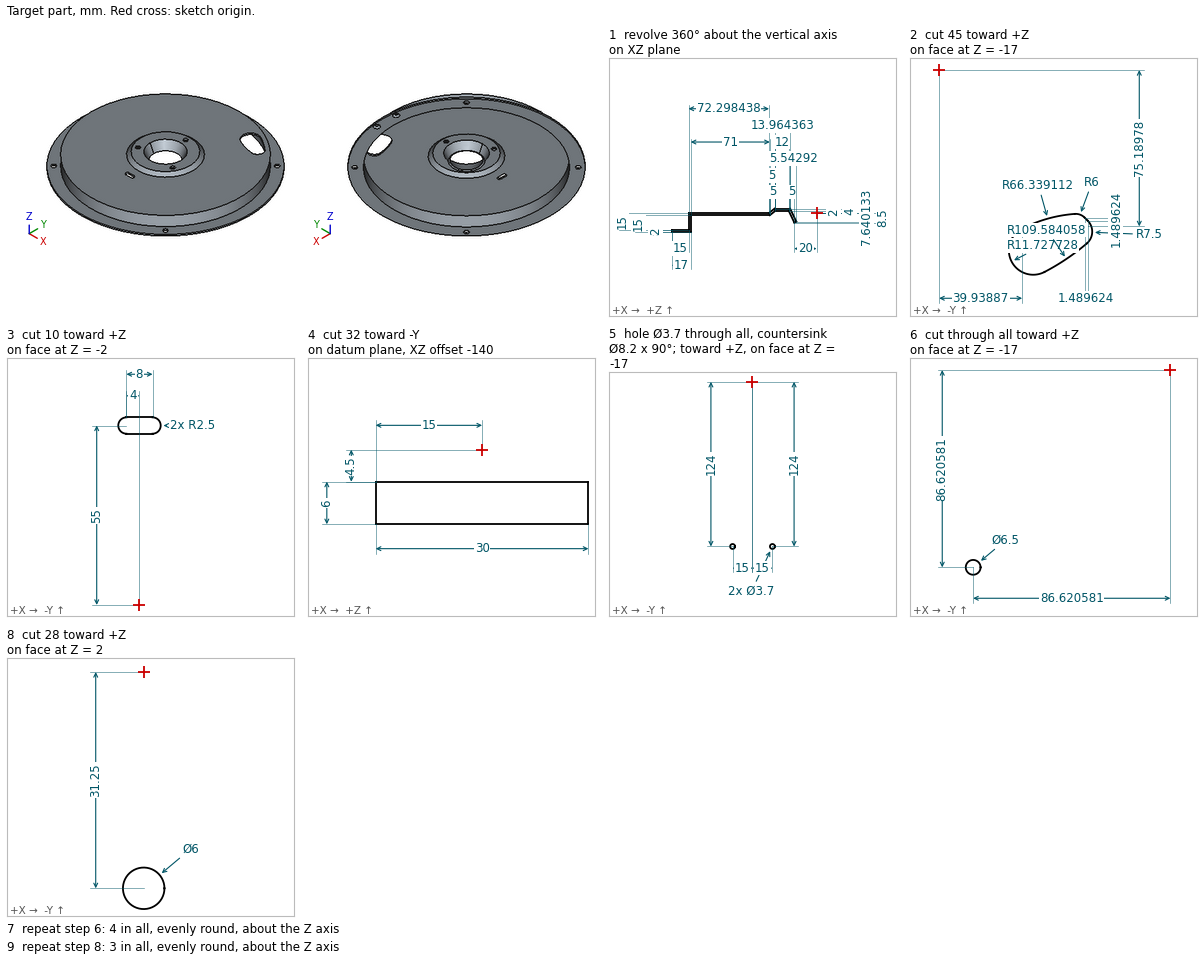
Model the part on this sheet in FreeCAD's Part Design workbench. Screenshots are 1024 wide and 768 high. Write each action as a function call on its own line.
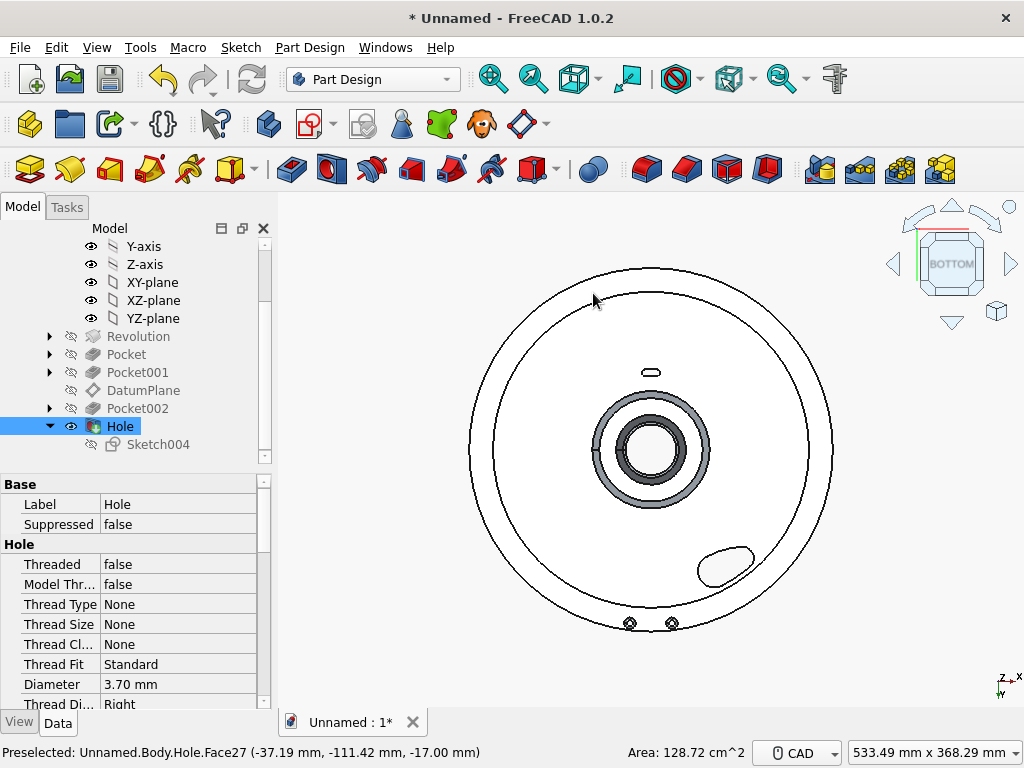
click(310, 124)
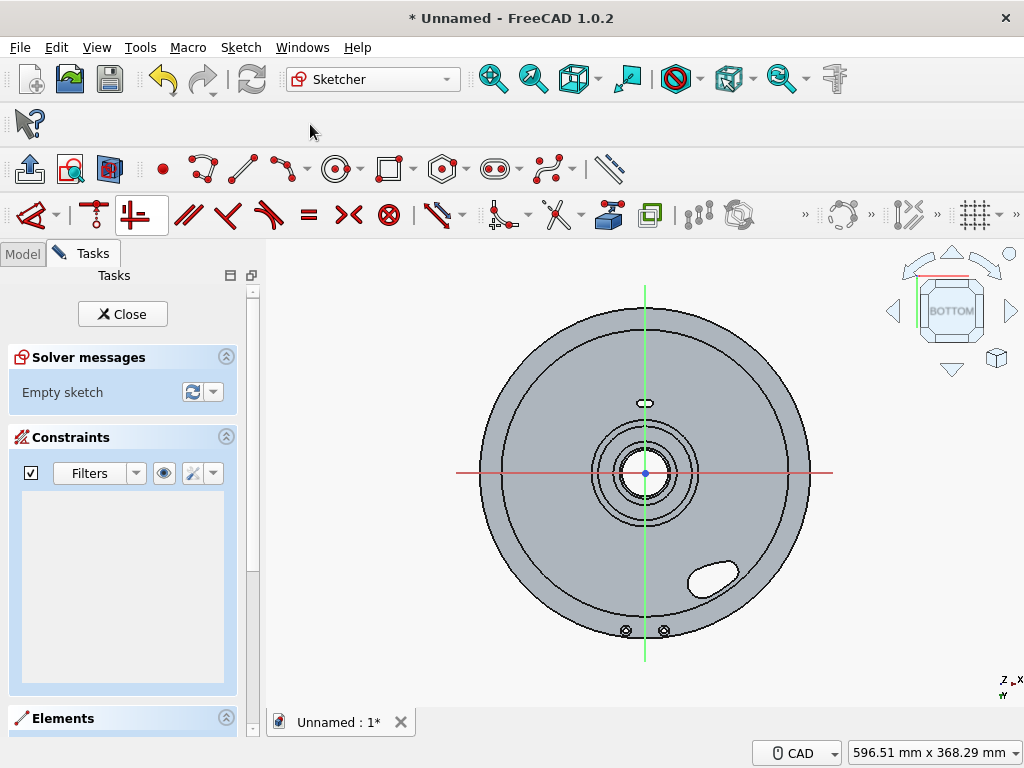
scroll(533, 589, up, 15)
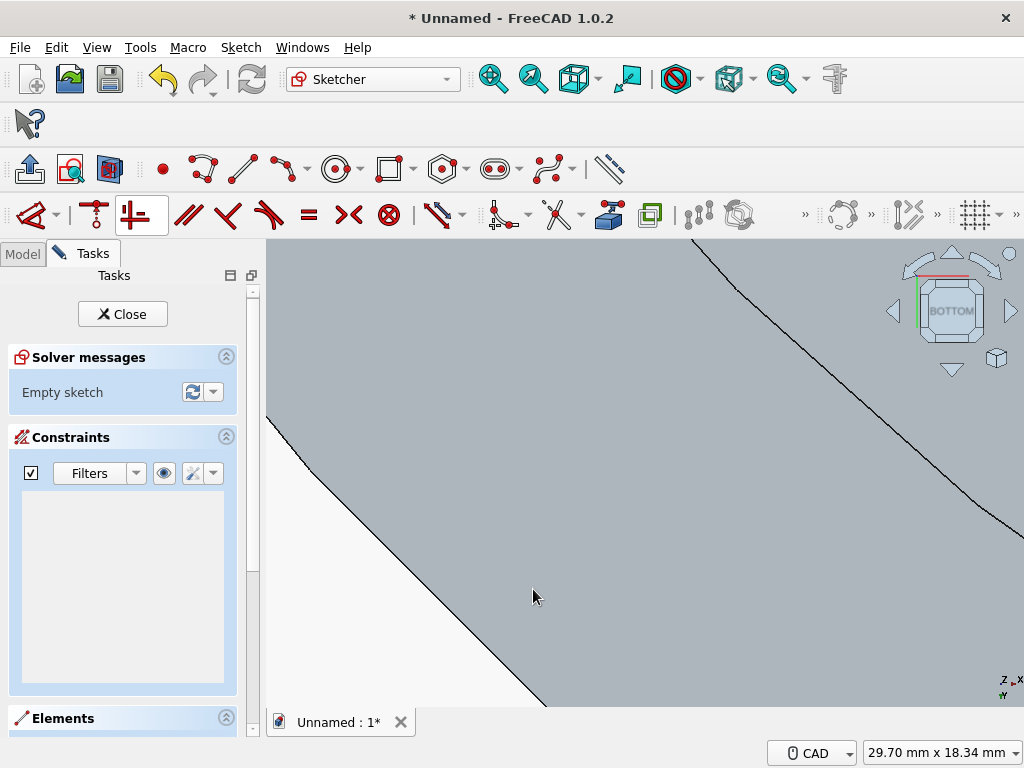
scroll(551, 447, up, 3)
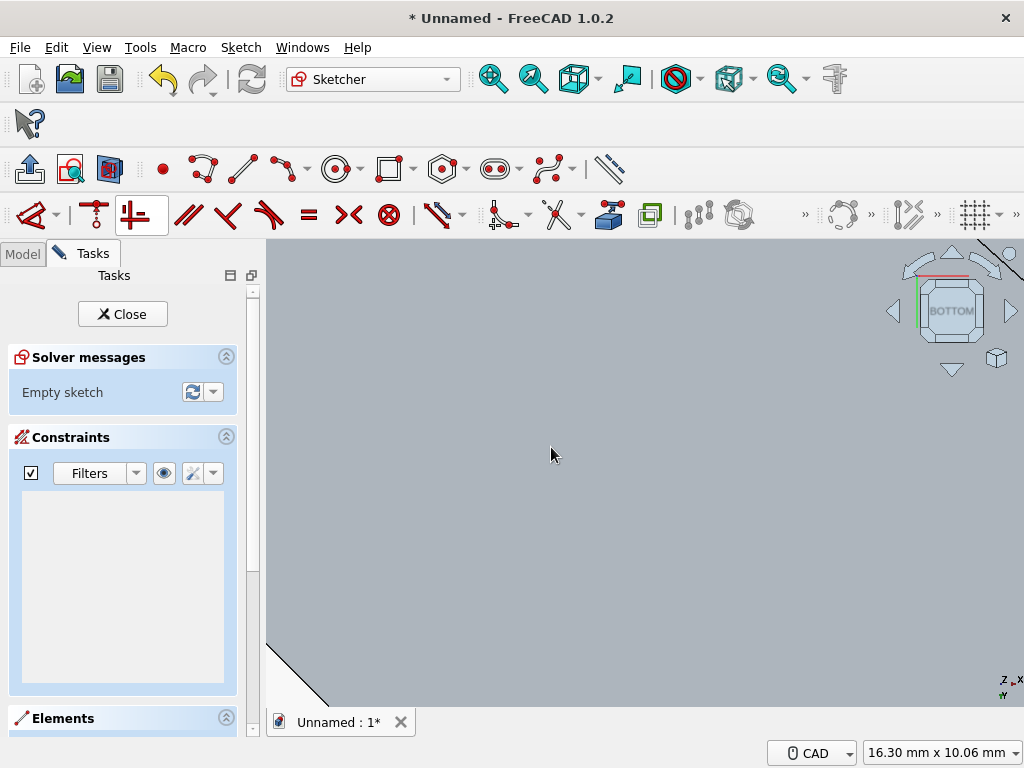
click(336, 170)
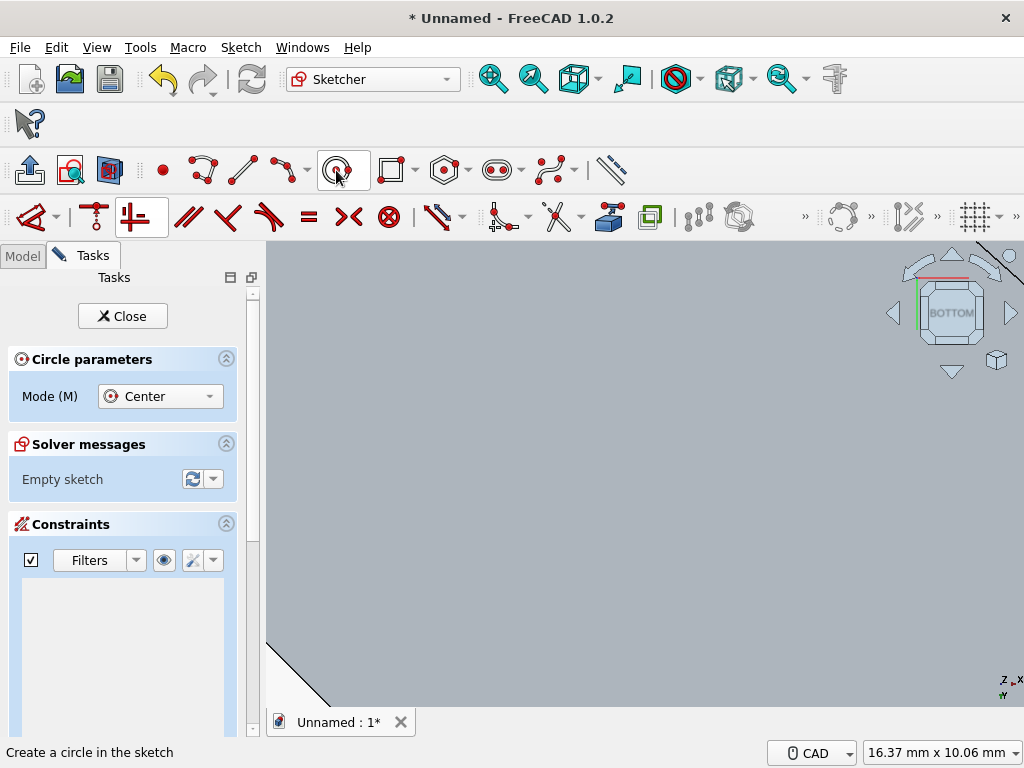
click(577, 473)
click(683, 367)
key(Escape)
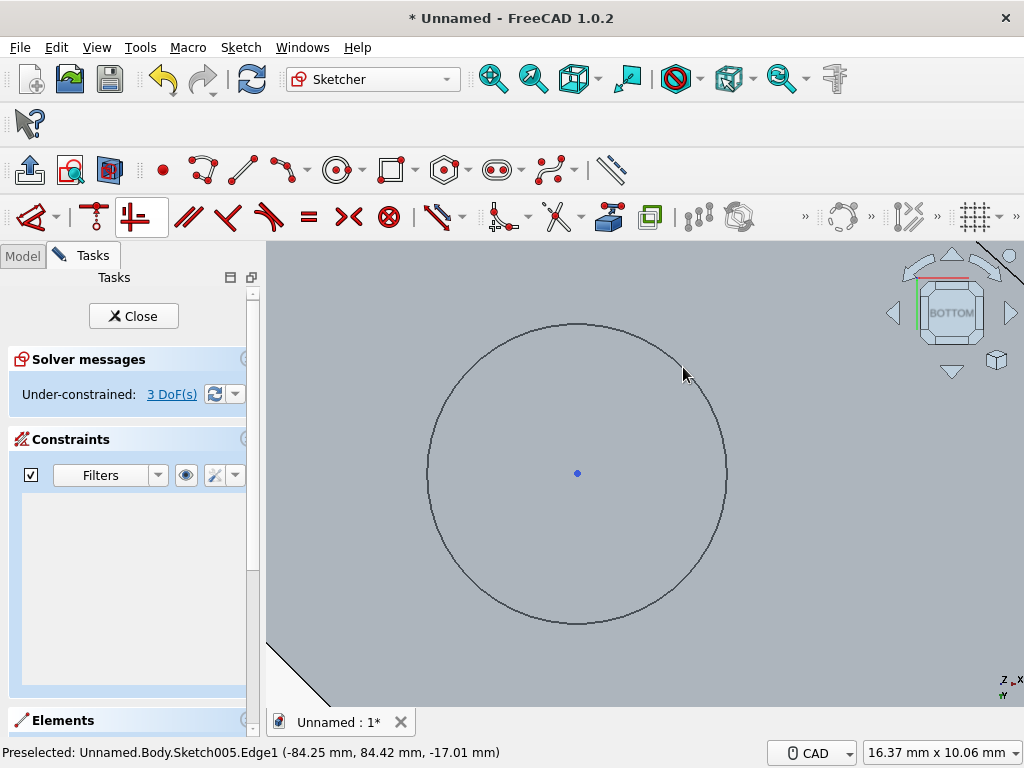
click(32, 218)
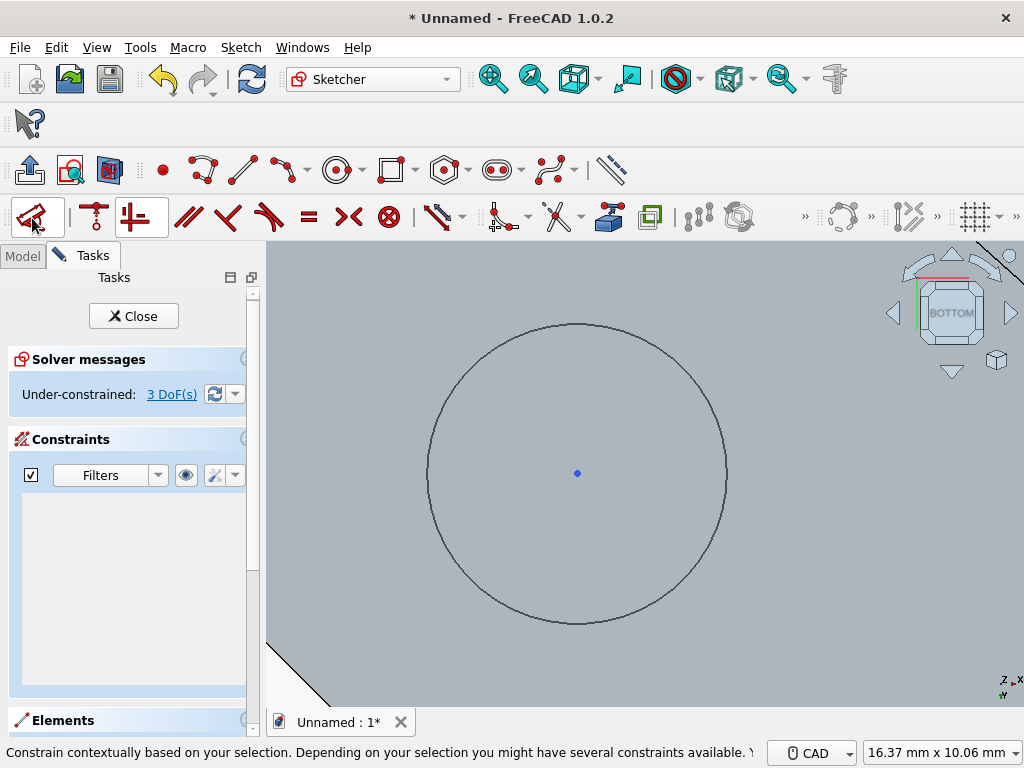
click(683, 368)
click(706, 345)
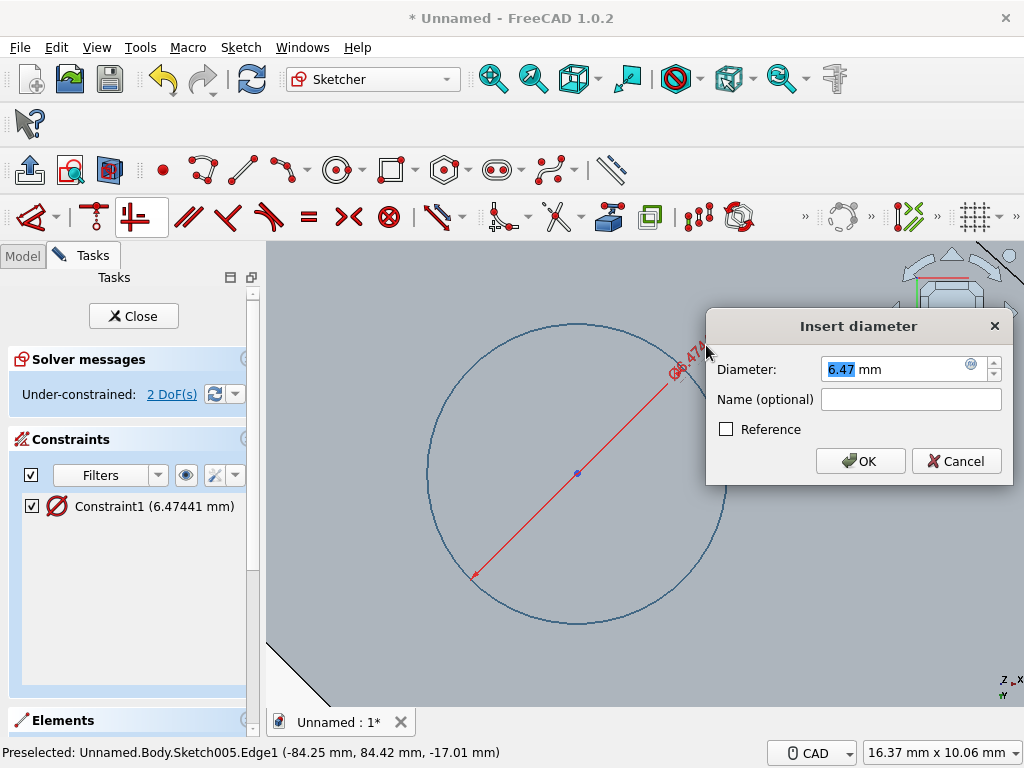
text(6.5)
key(Return)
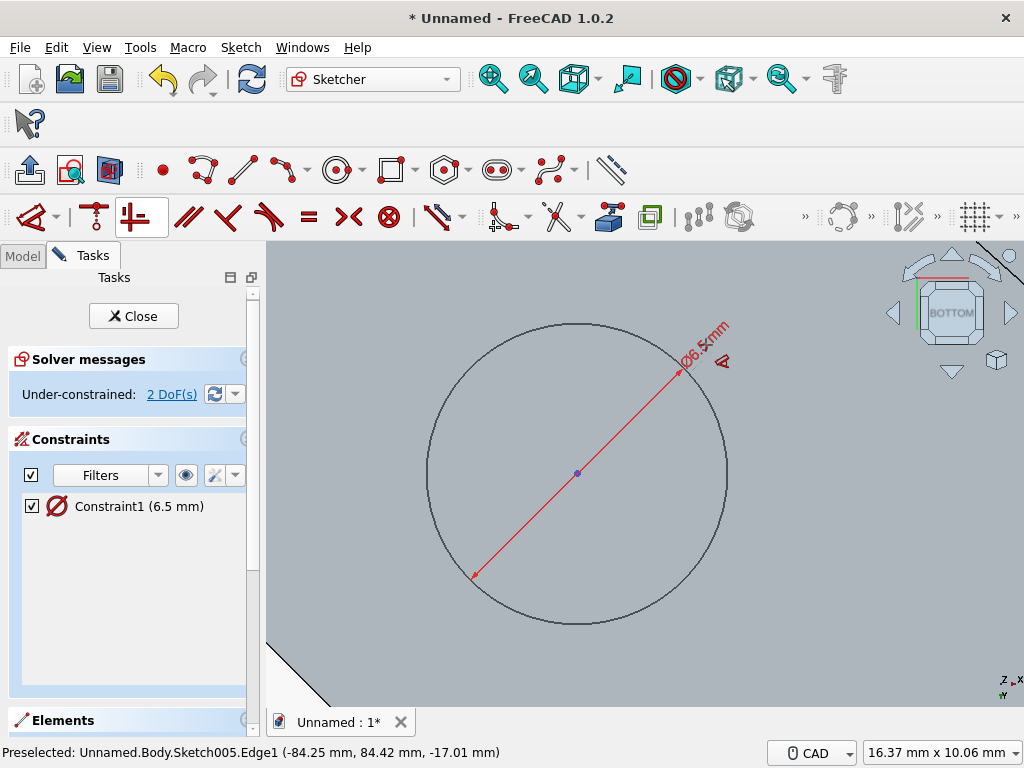
click(577, 474)
click(653, 508)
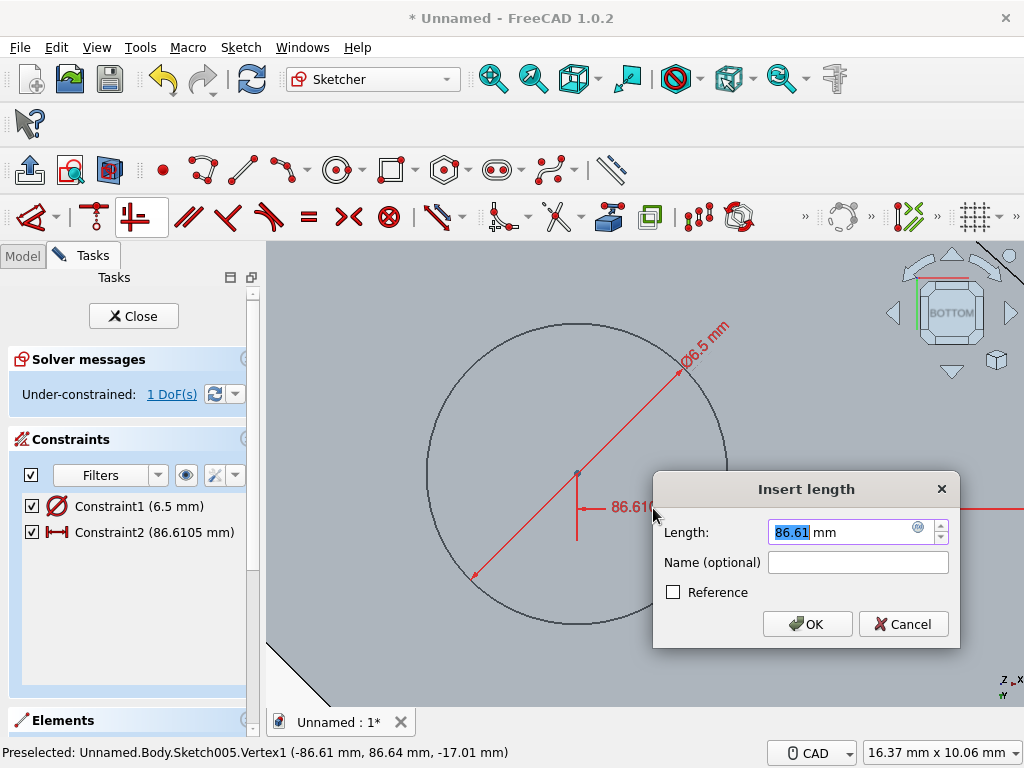
text(86.620581)
key(Return)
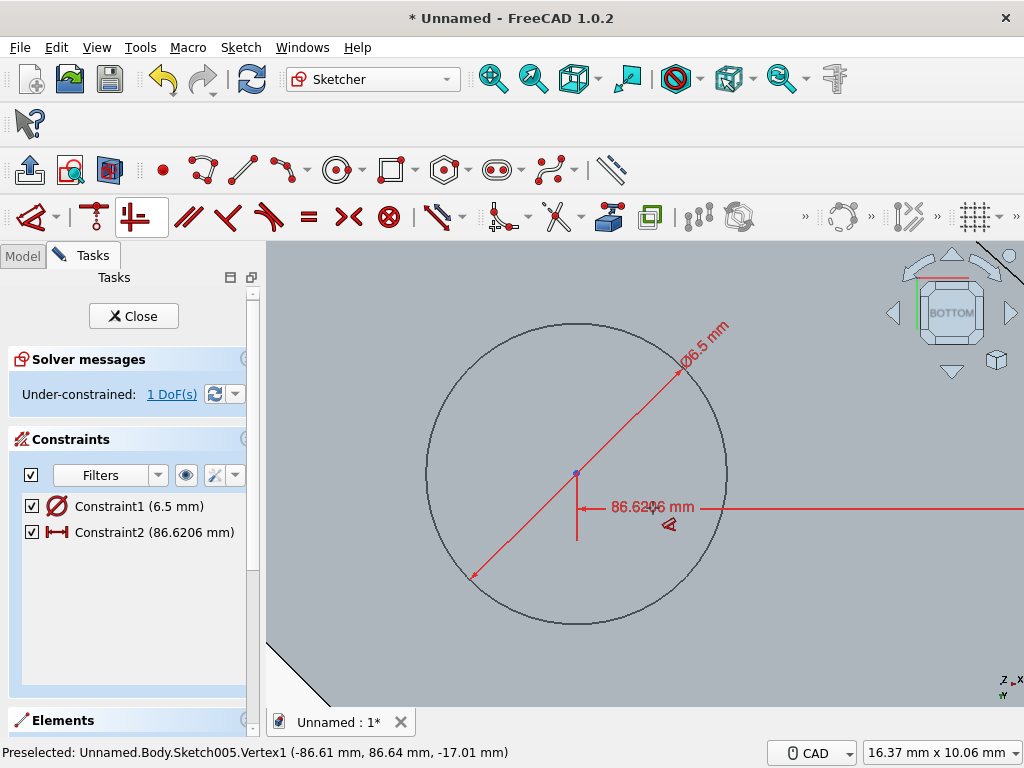
click(577, 474)
click(543, 371)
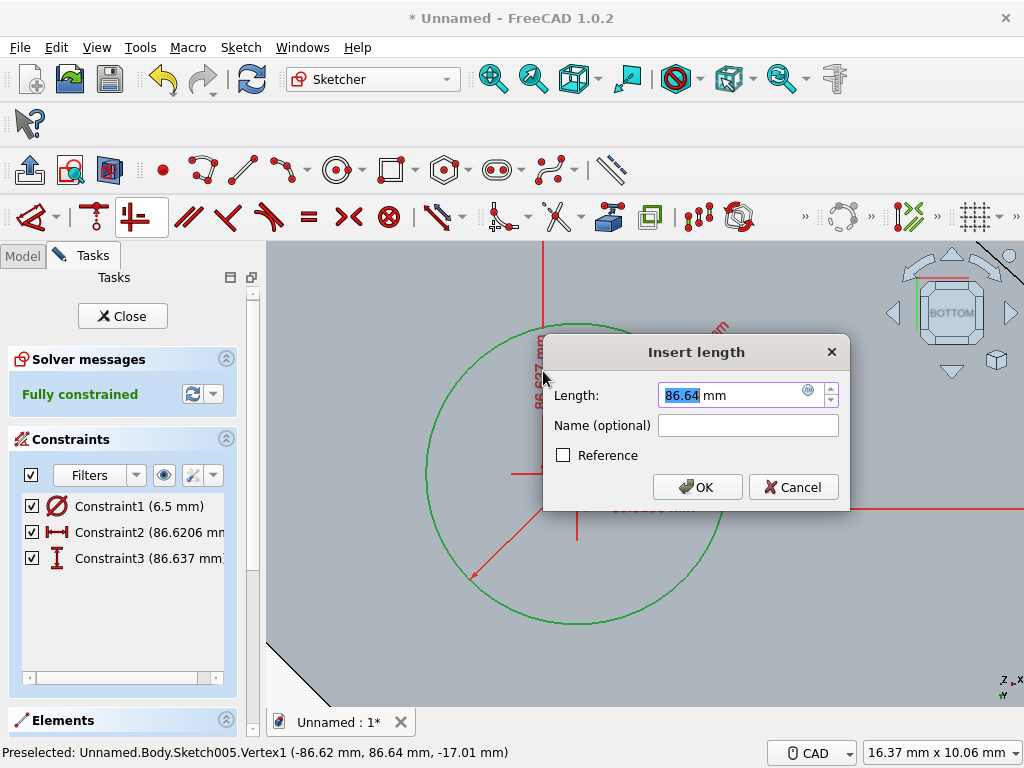
text(86.620581)
key(Return)
key(Escape)